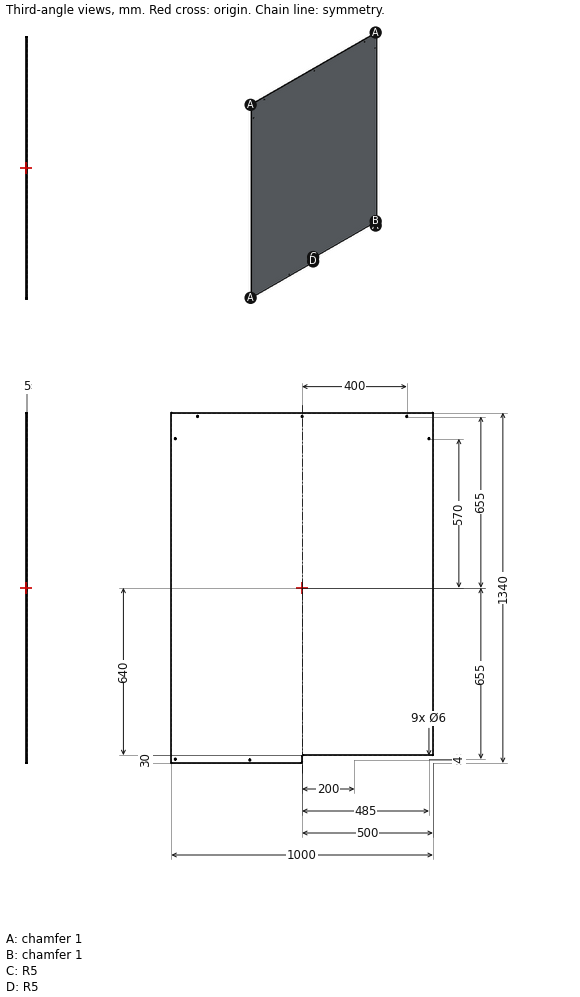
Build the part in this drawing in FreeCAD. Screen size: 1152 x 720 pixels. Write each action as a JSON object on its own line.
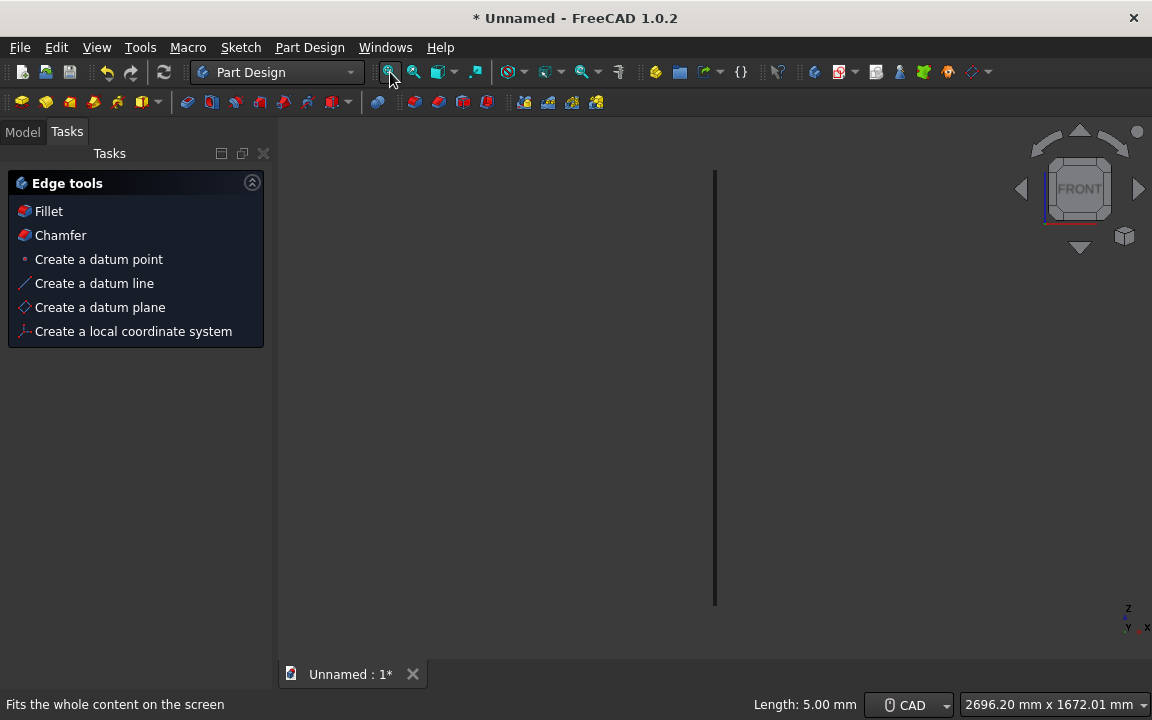
{"action": "scroll", "coordinate": [715, 604], "scroll_direction": "up", "scroll_amount": 15}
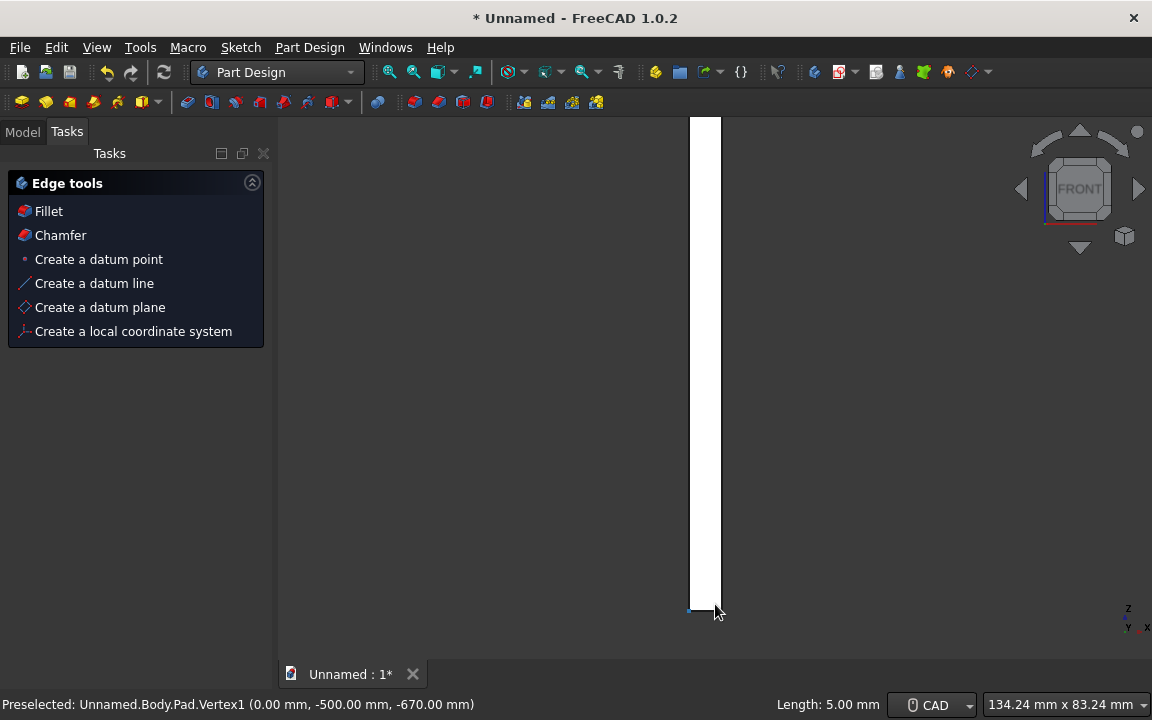
{"action": "left_click", "coordinate": [705, 610], "text": "ctrl"}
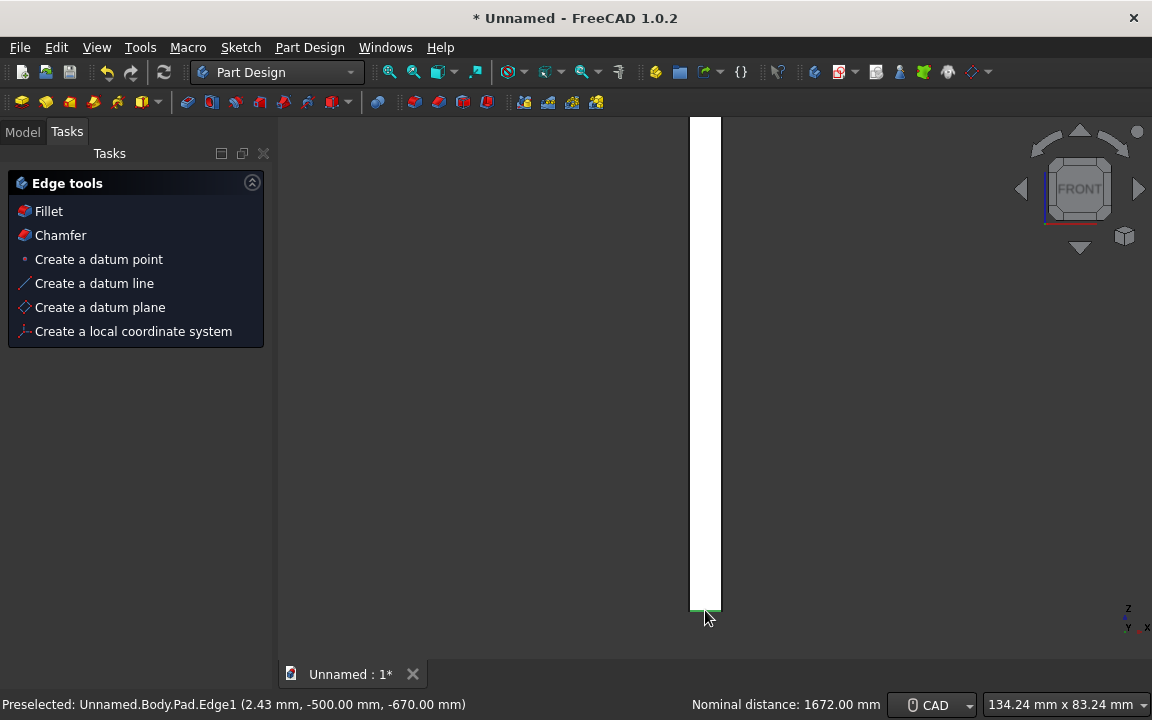
{"action": "left_click", "coordinate": [390, 72]}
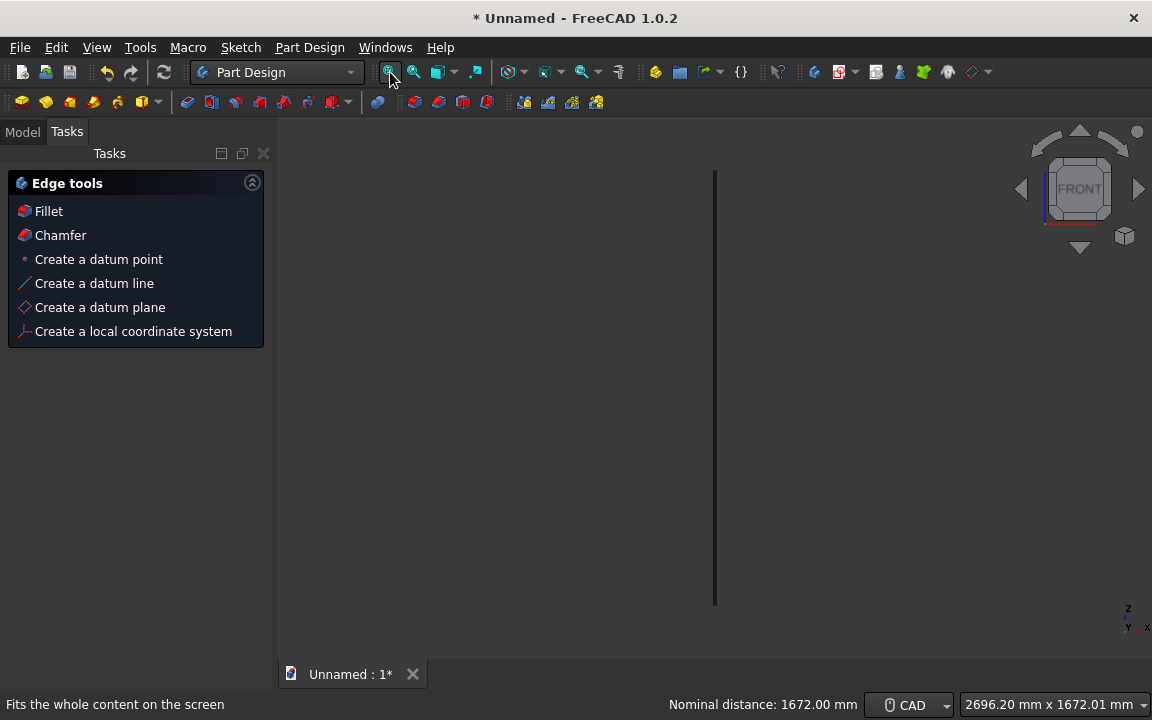
{"action": "key", "text": "3"}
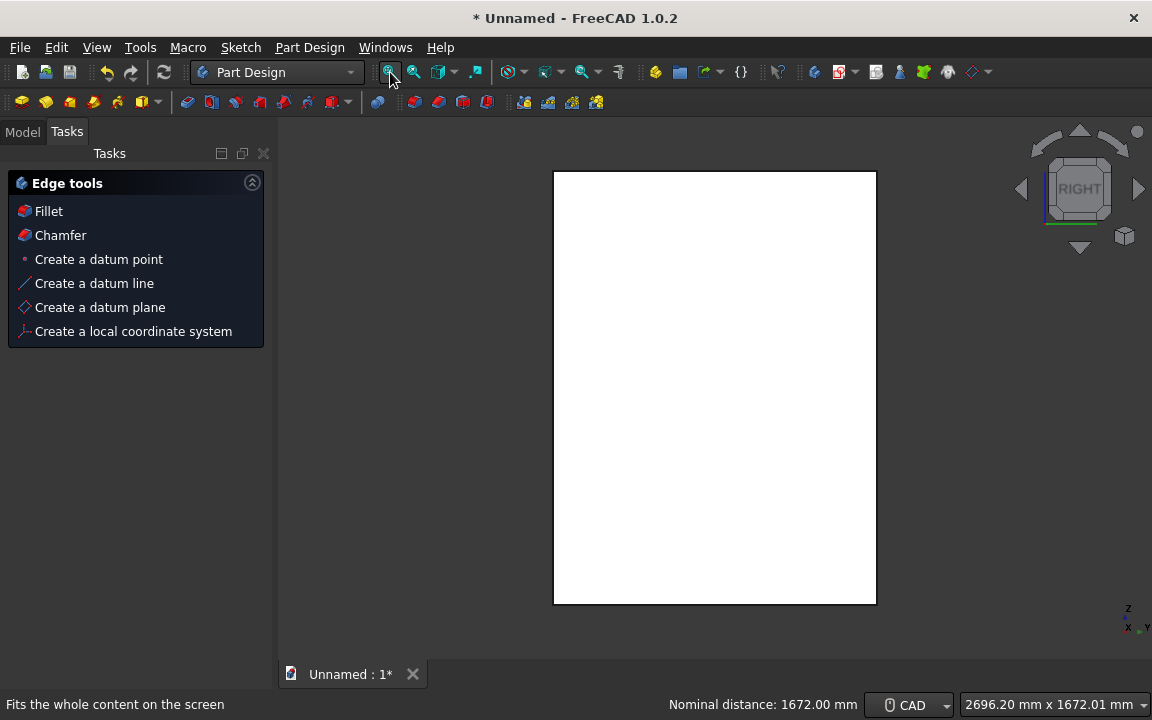
{"action": "scroll", "coordinate": [877, 604], "scroll_direction": "up", "scroll_amount": 15}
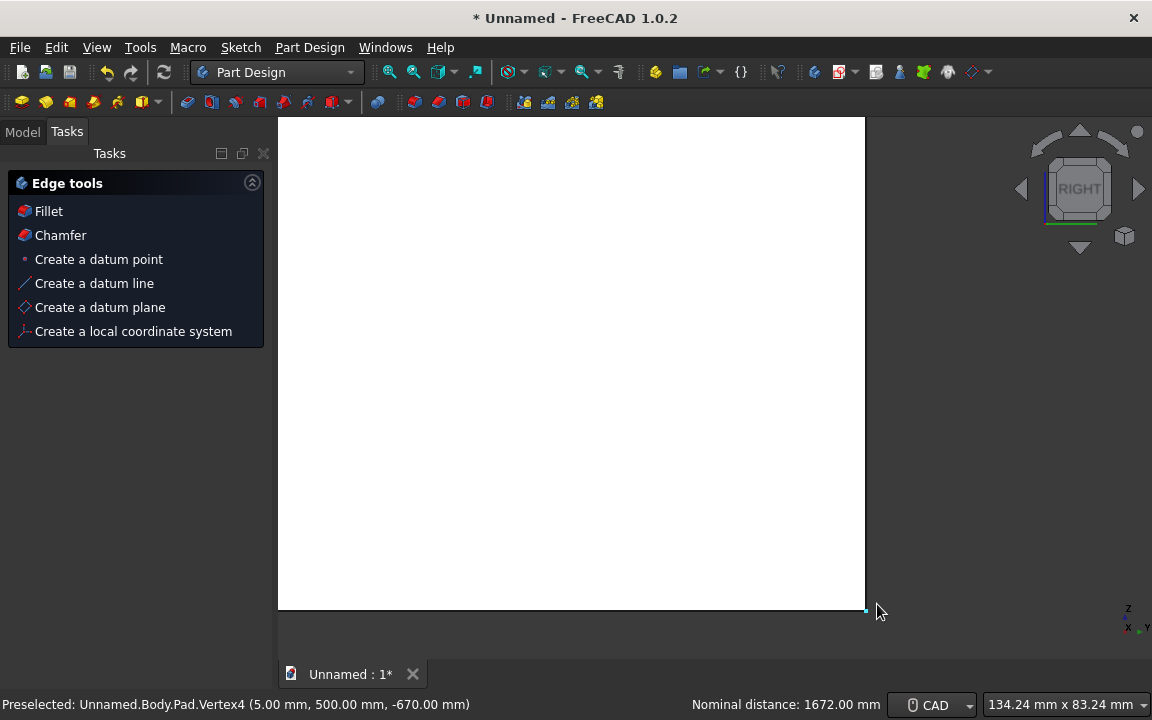
{"action": "left_click", "coordinate": [390, 72]}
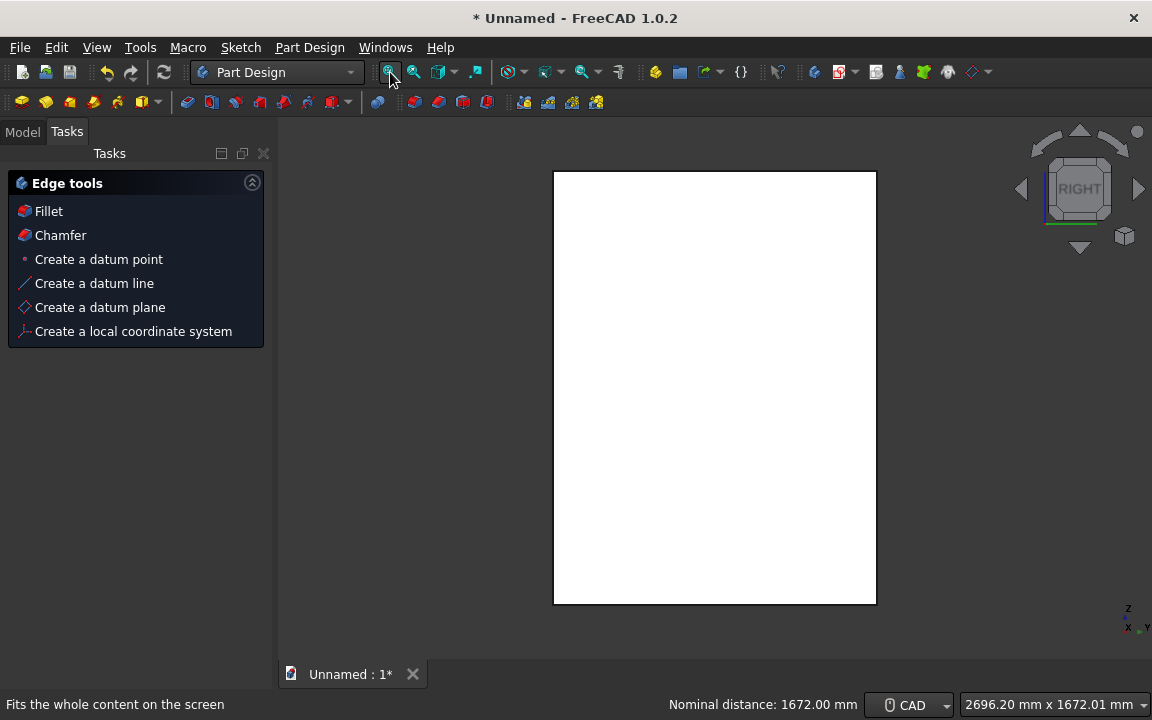
{"action": "key", "text": "5"}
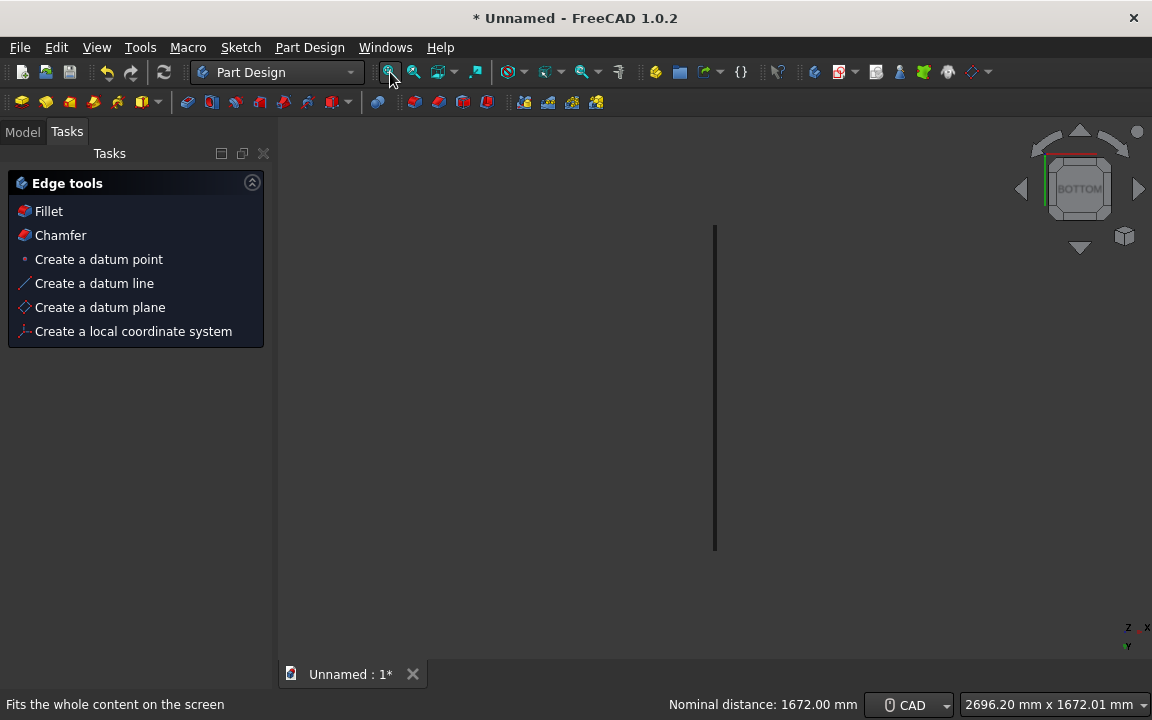
{"action": "scroll", "coordinate": [715, 549], "scroll_direction": "up", "scroll_amount": 15}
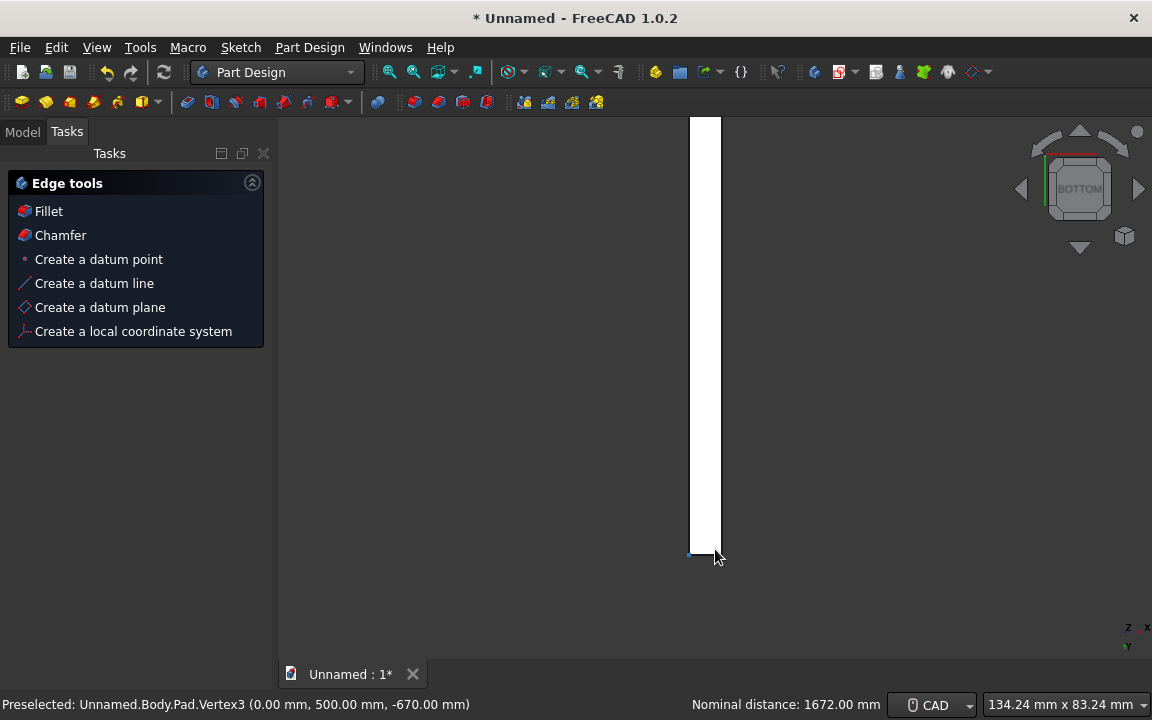
{"action": "left_click", "coordinate": [705, 554], "text": "ctrl"}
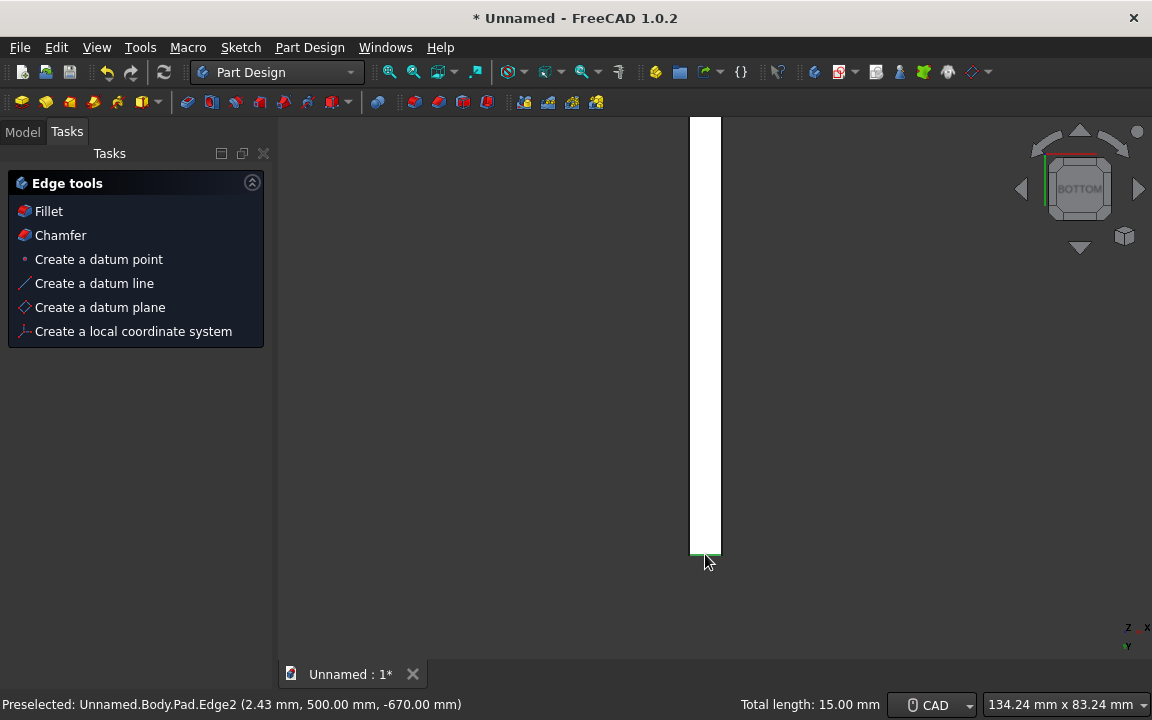
{"action": "left_click", "coordinate": [390, 72]}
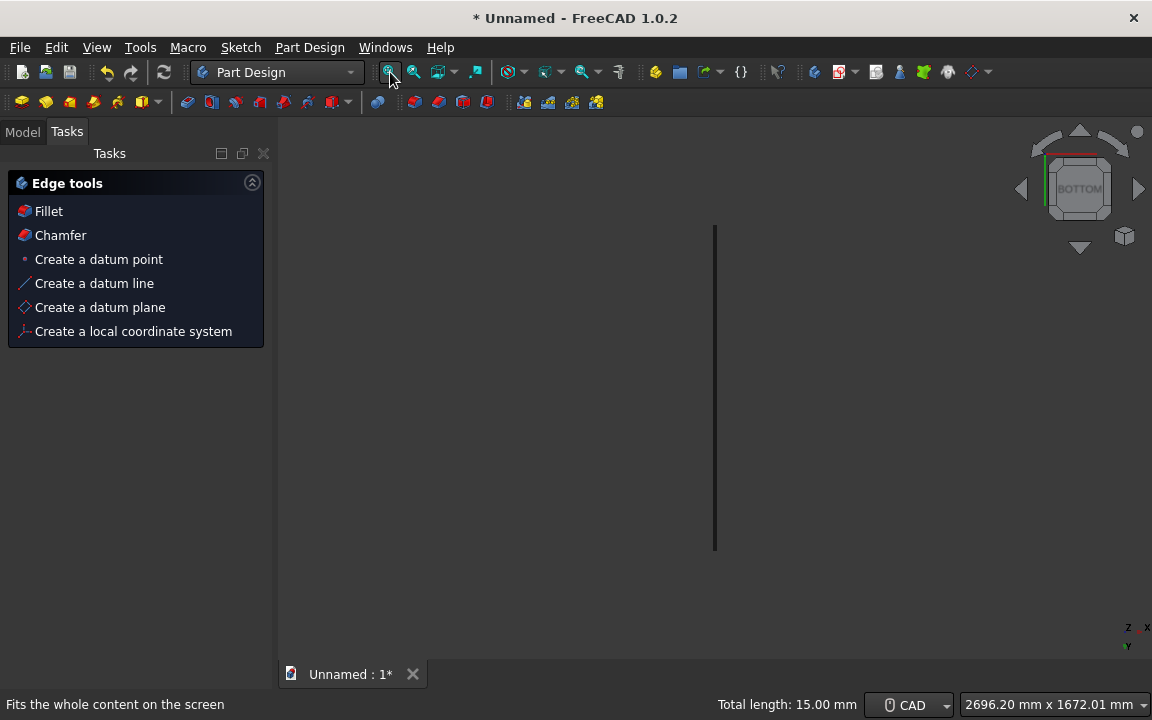
{"action": "key", "text": "4"}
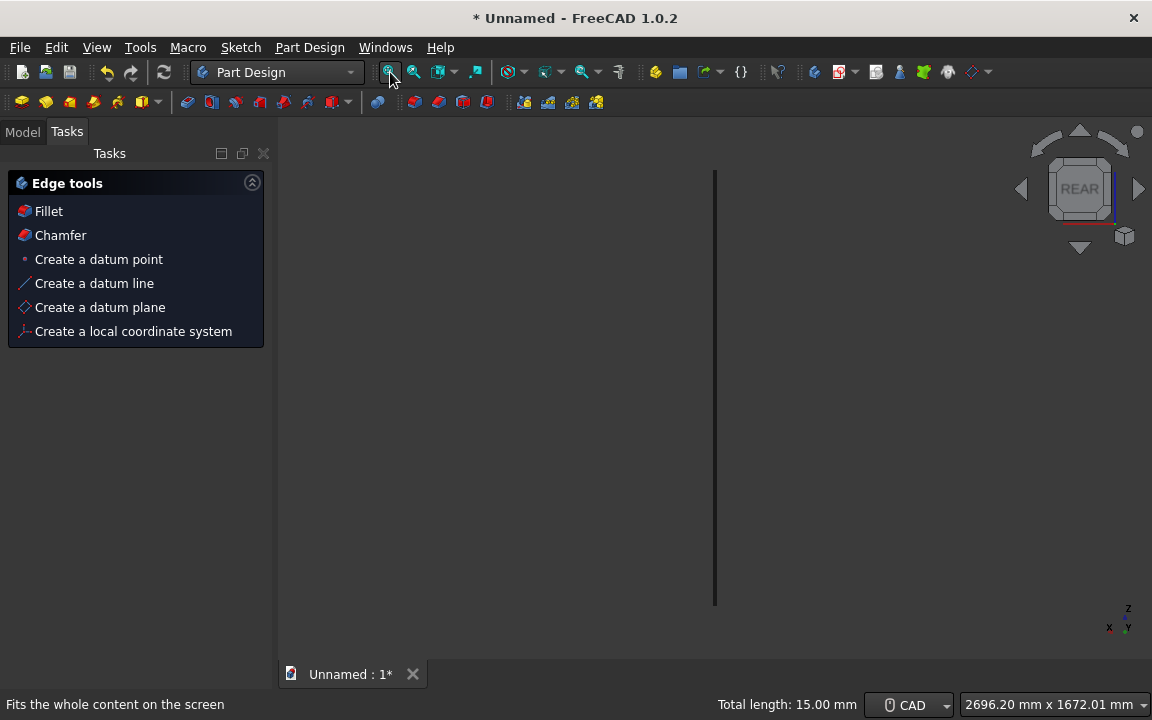
{"action": "scroll", "coordinate": [715, 170], "scroll_direction": "up", "scroll_amount": 15}